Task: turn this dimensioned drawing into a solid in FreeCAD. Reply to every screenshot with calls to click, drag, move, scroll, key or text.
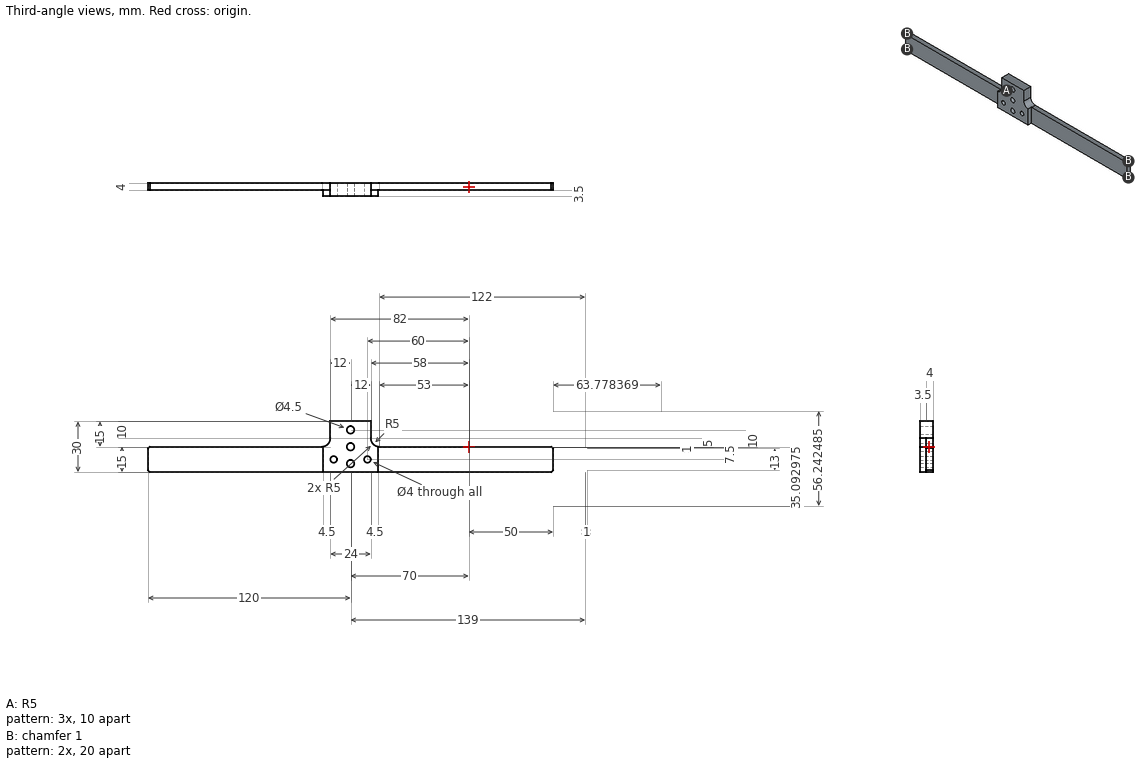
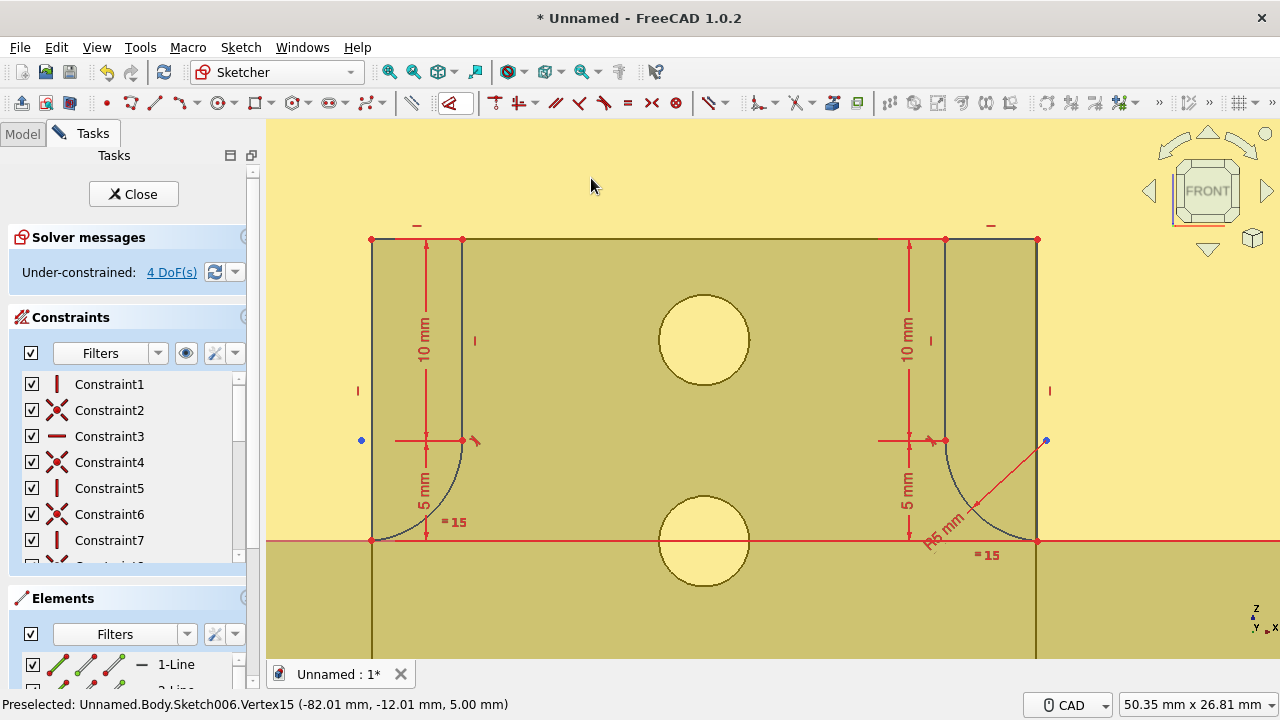
click(973, 239)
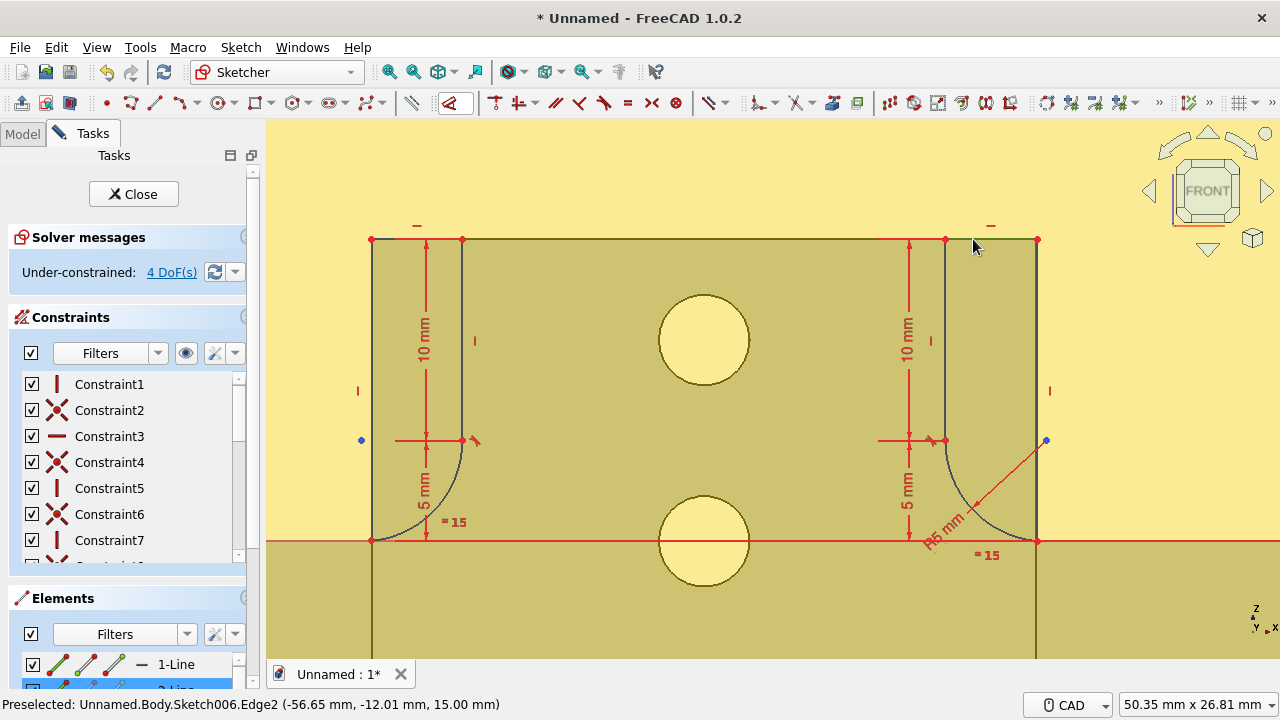
click(468, 104)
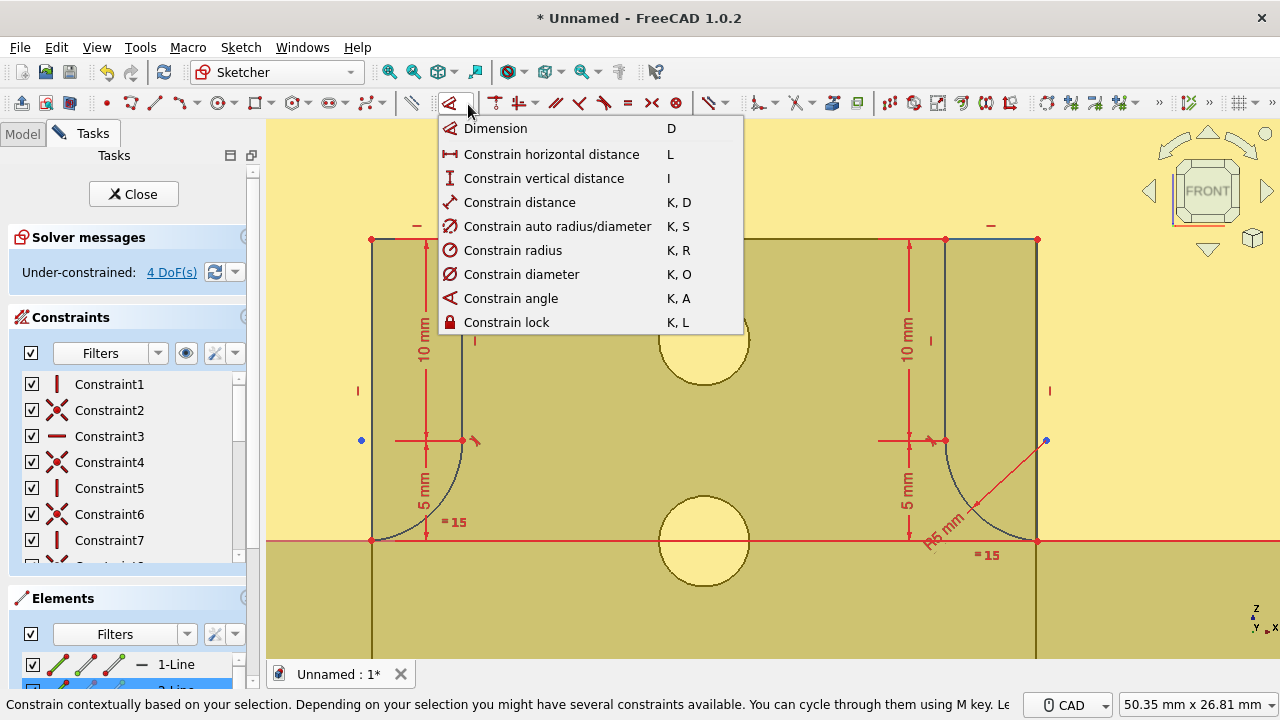
click(591, 154)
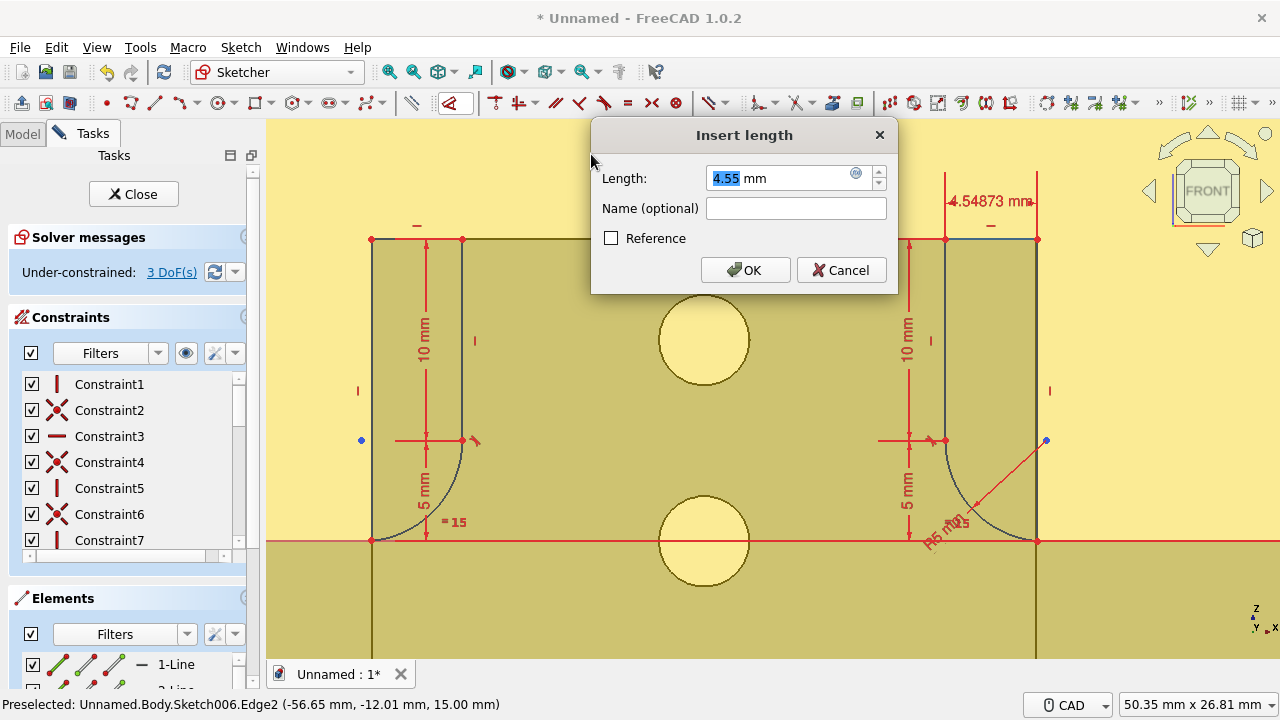
text(4.5)
key(Return)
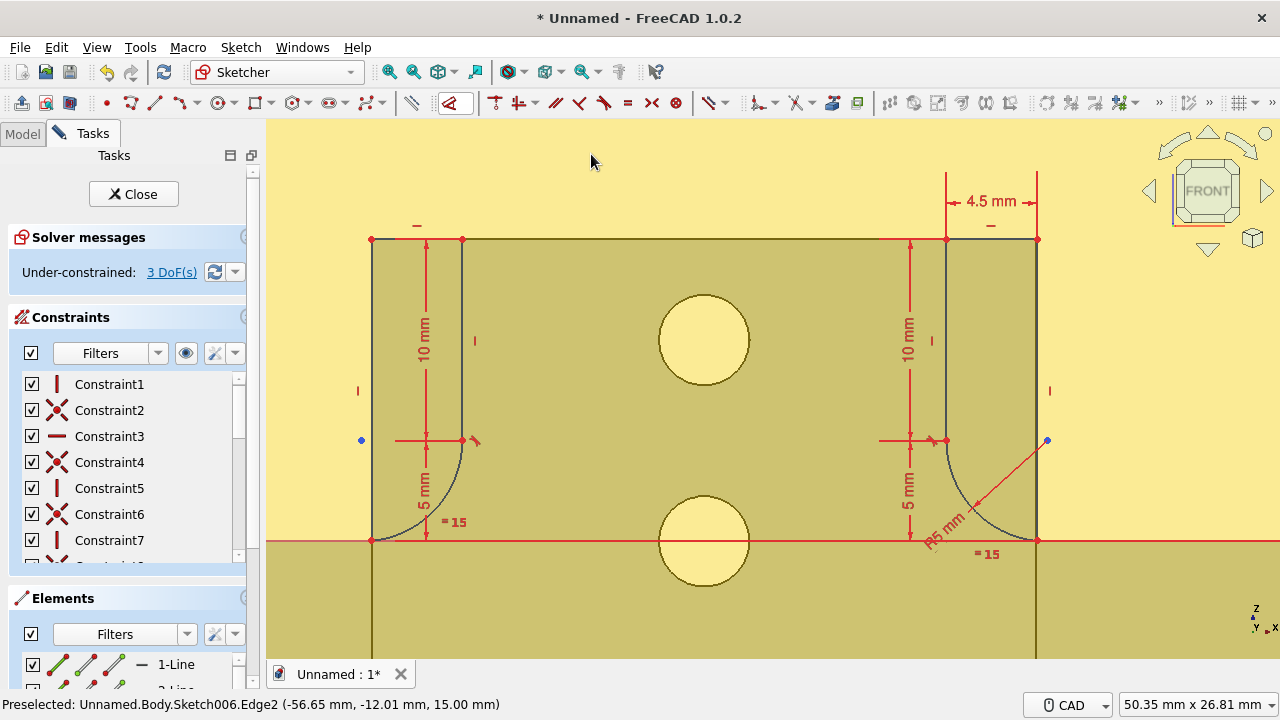
click(399, 239)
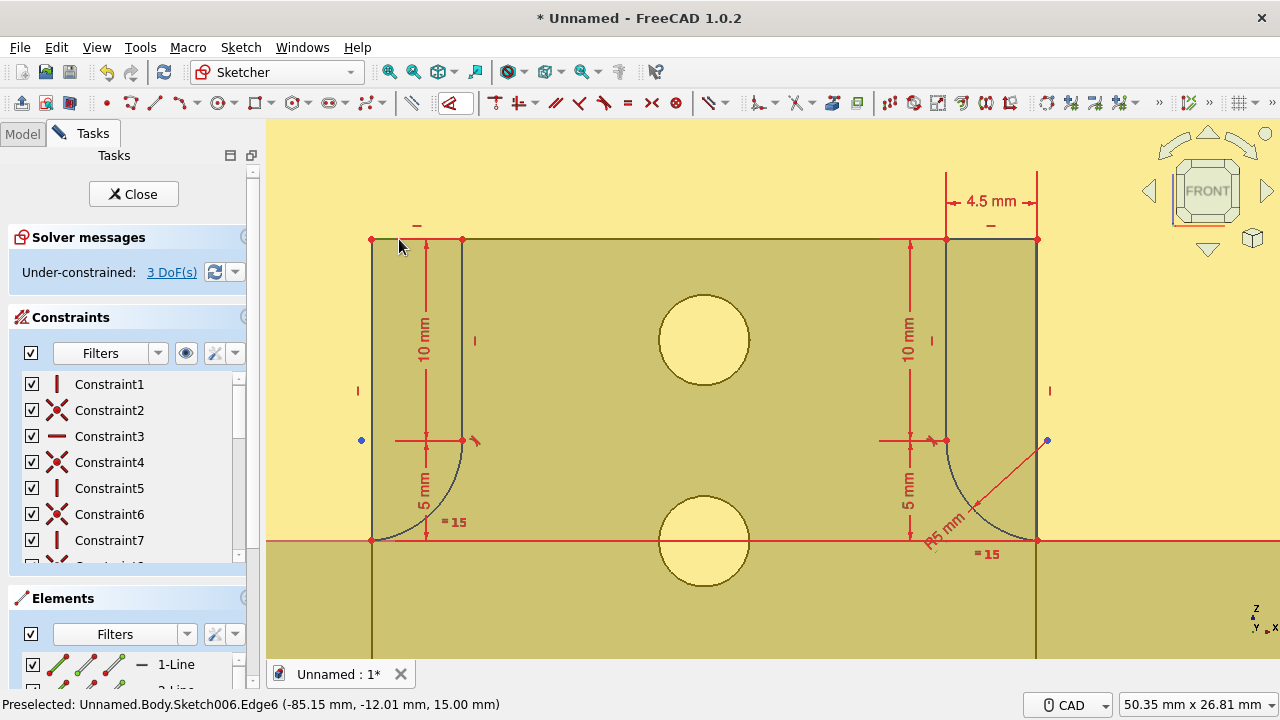
click(468, 104)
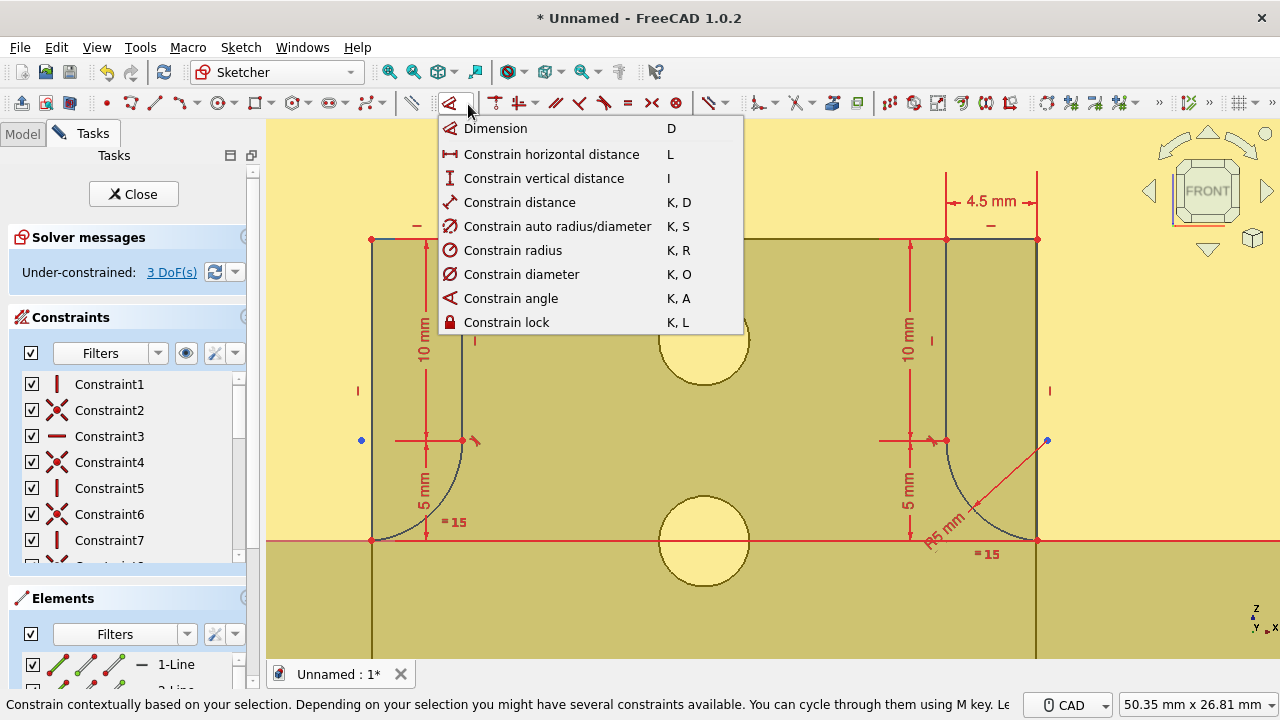
click(591, 154)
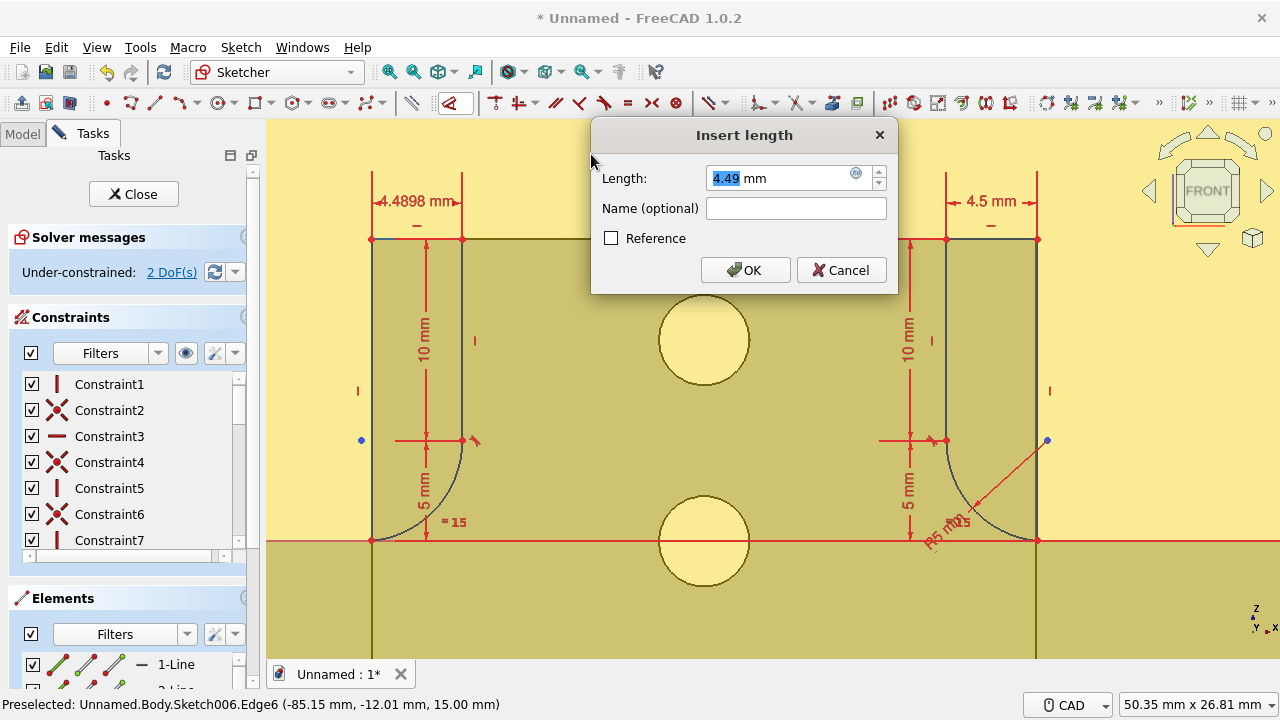
text(4.5)
key(Return)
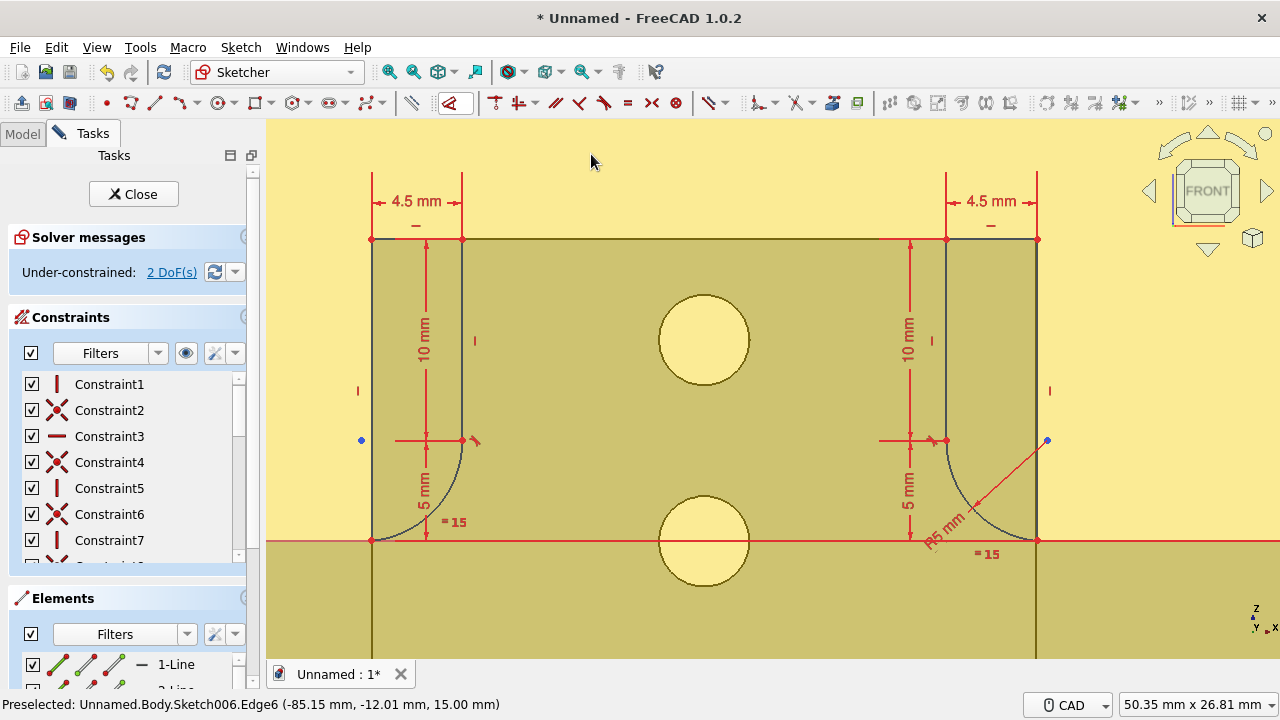
click(946, 441)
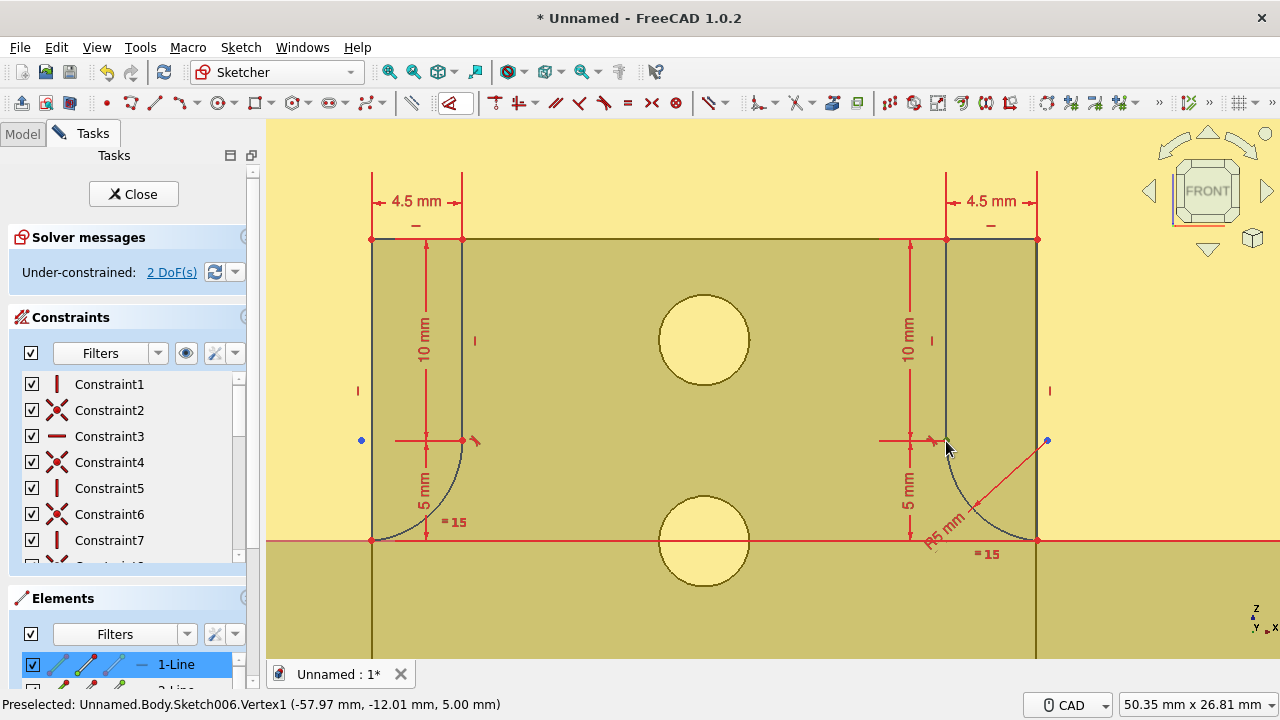
click(468, 104)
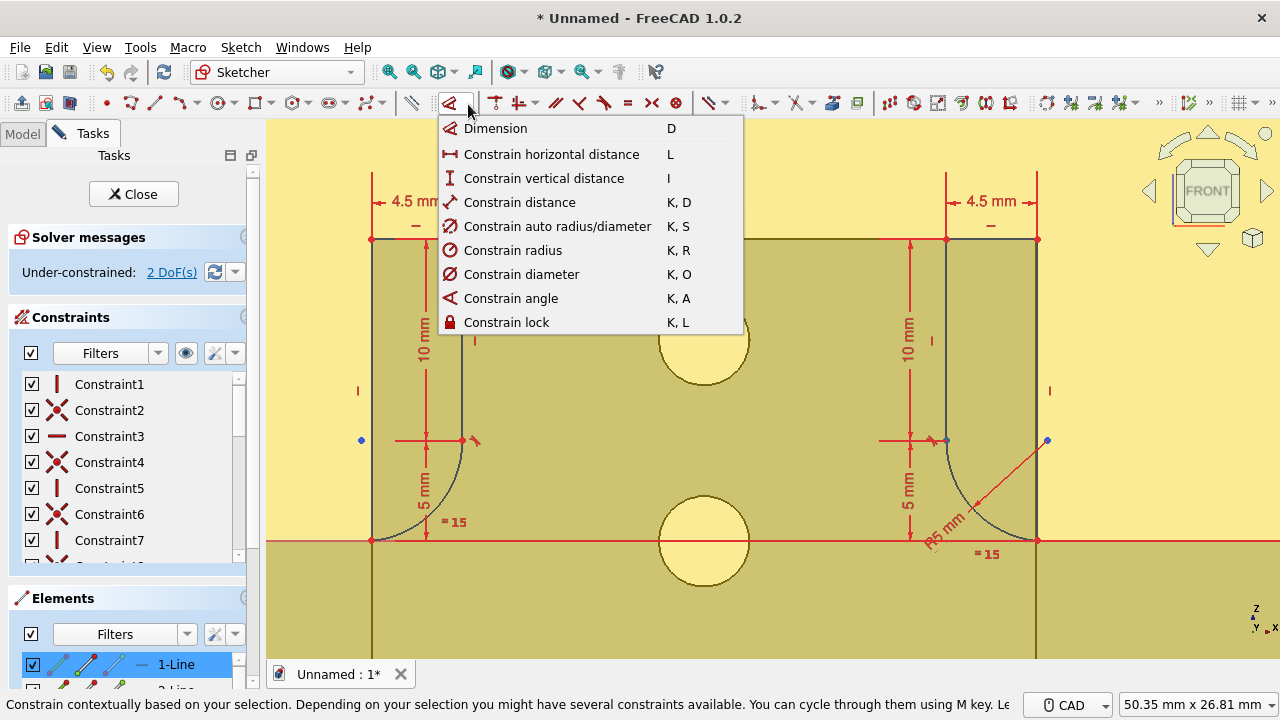
click(591, 154)